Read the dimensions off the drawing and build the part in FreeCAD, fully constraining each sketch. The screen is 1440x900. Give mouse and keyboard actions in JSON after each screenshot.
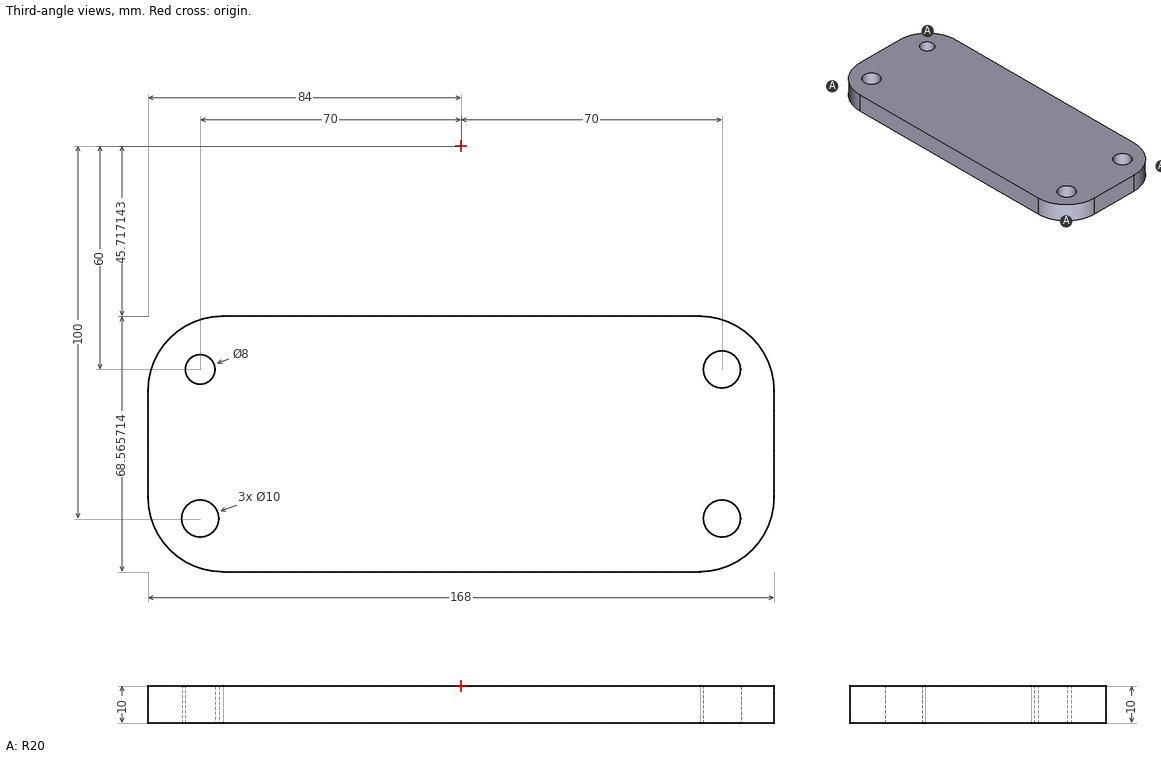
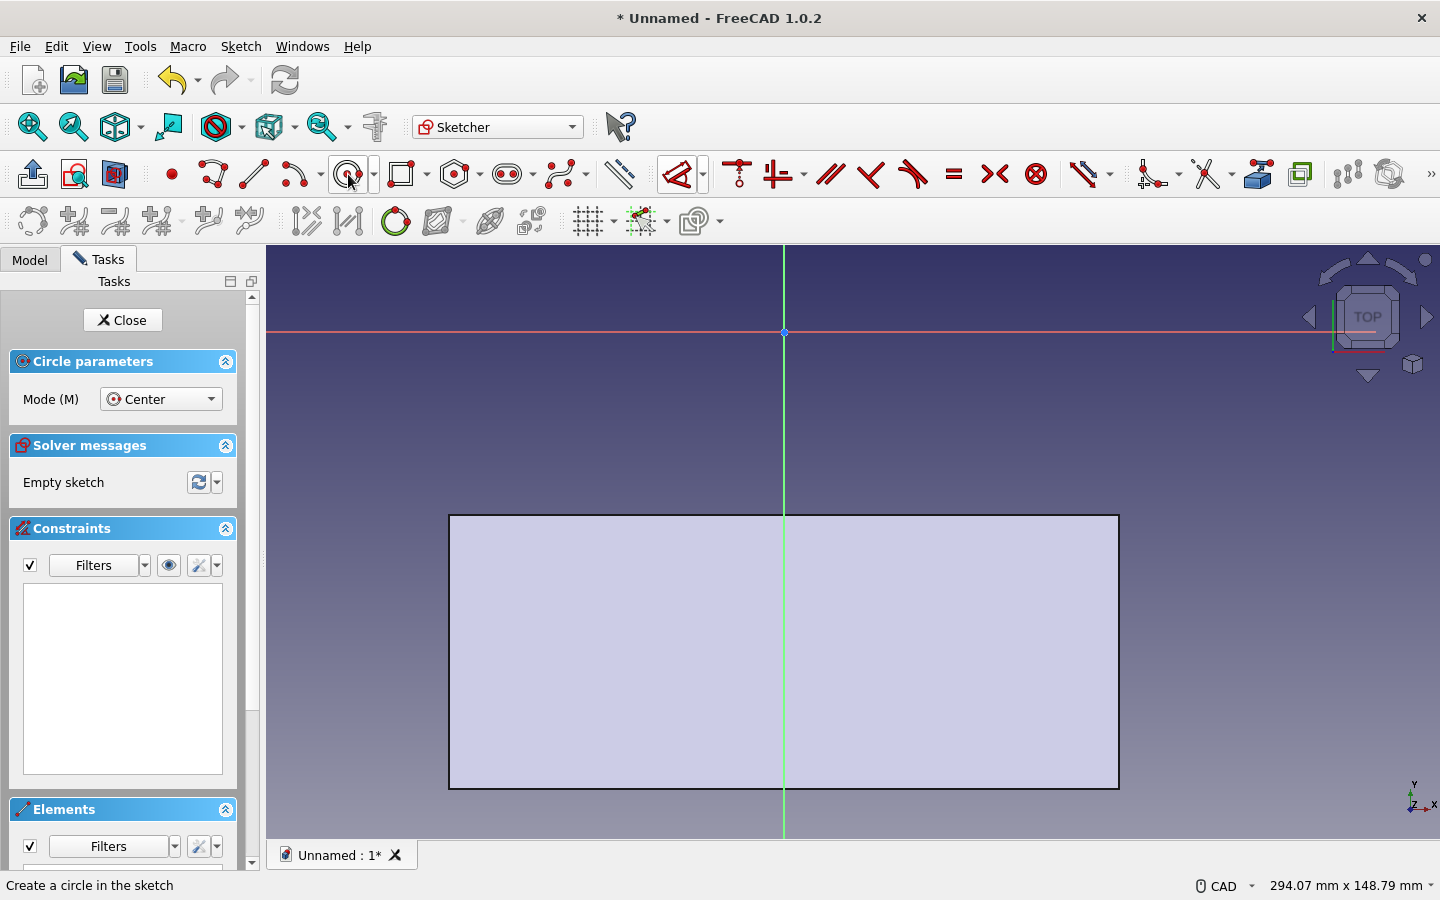
{"action": "scroll", "coordinate": [505, 572], "scroll_direction": "up", "scroll_amount": 2}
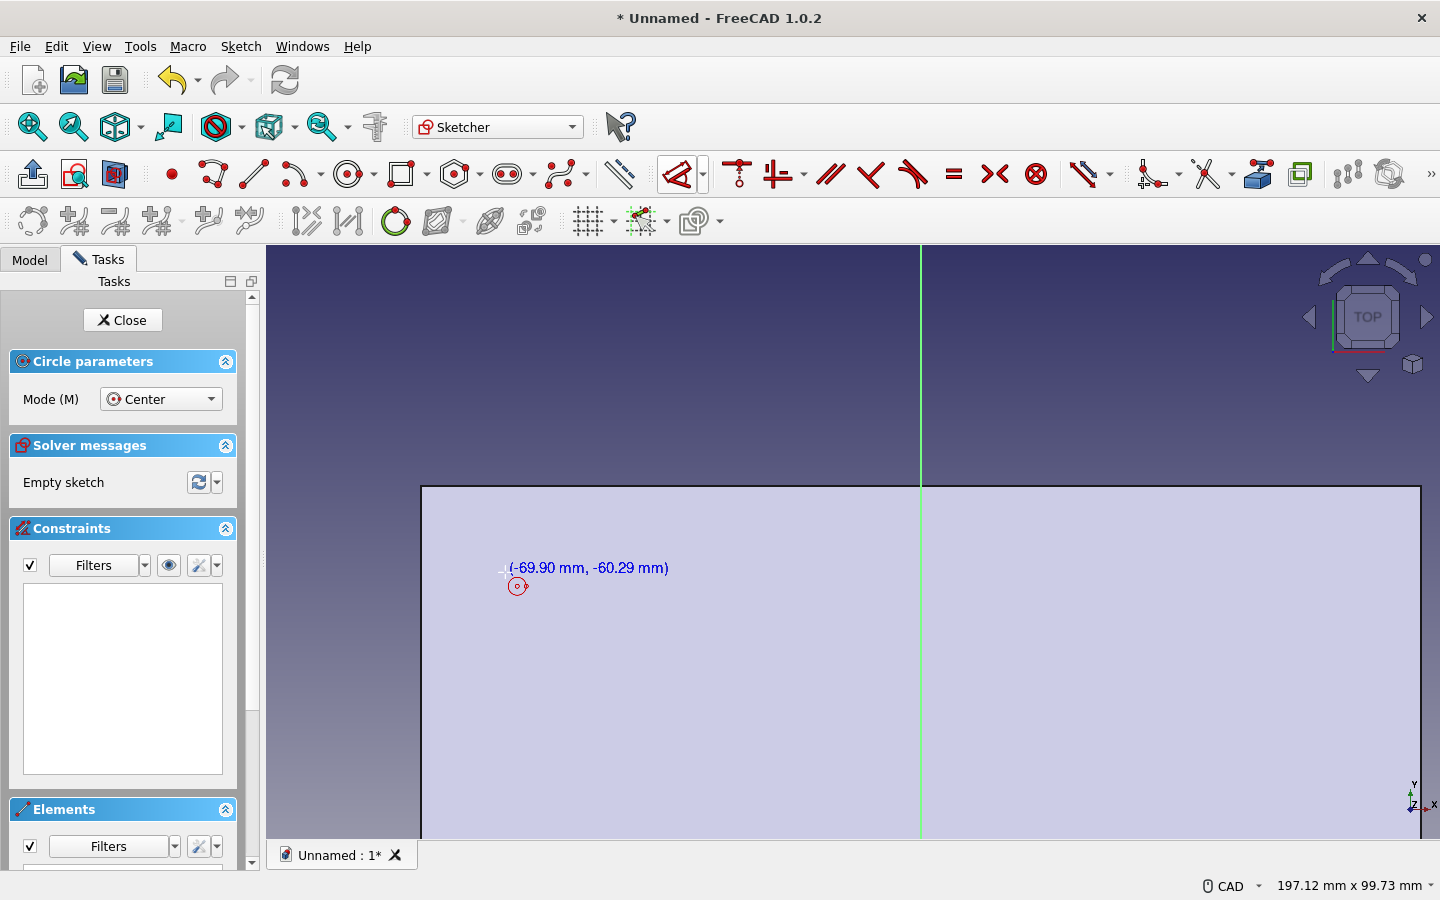
{"action": "left_click", "coordinate": [504, 572]}
{"action": "left_click", "coordinate": [521, 555]}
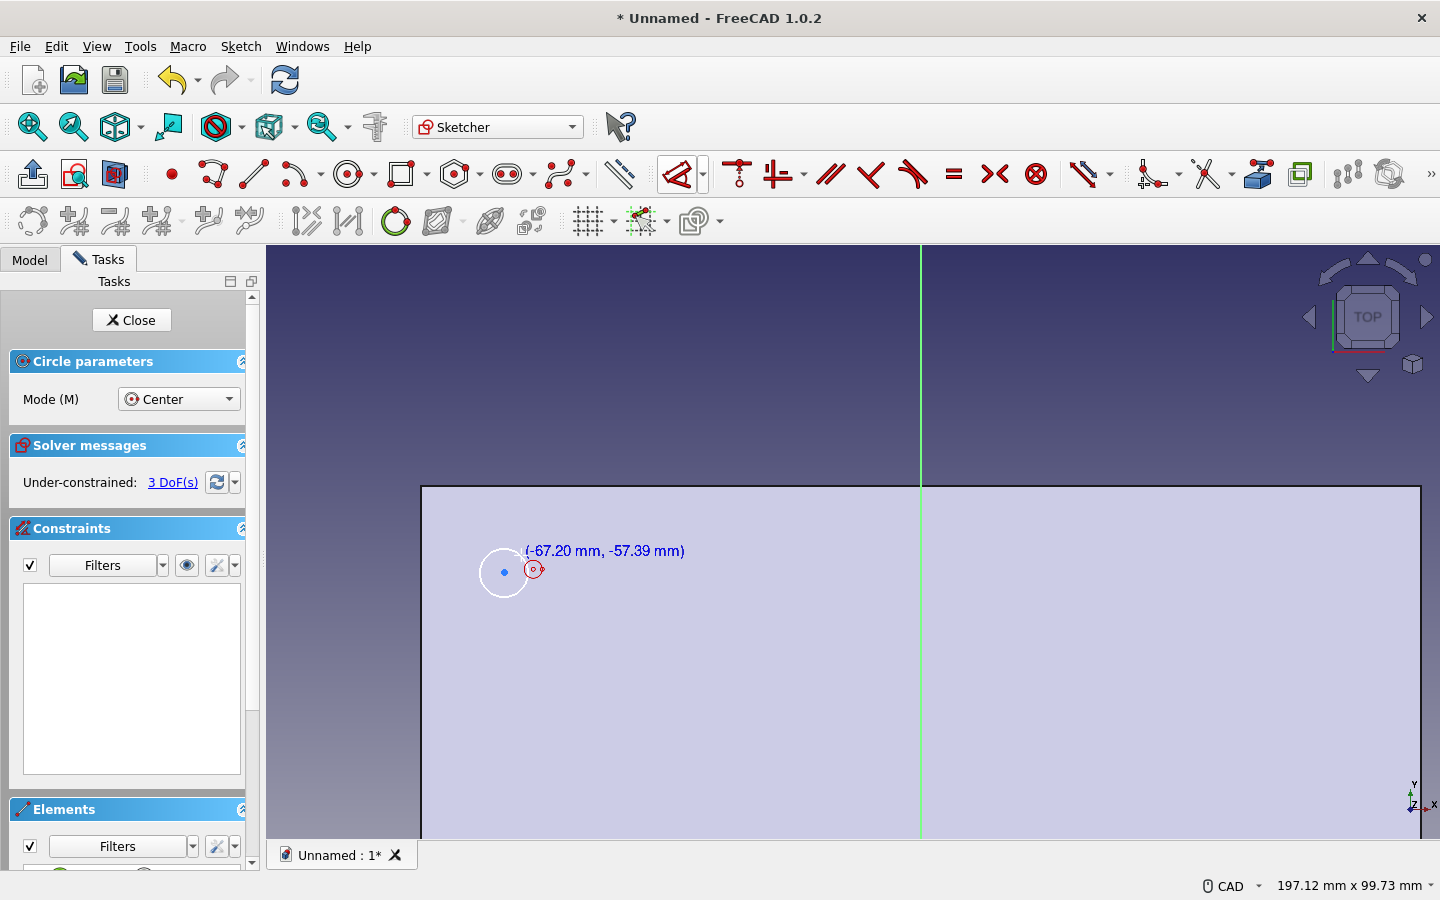
{"action": "left_click", "coordinate": [504, 810]}
{"action": "left_click", "coordinate": [525, 789]}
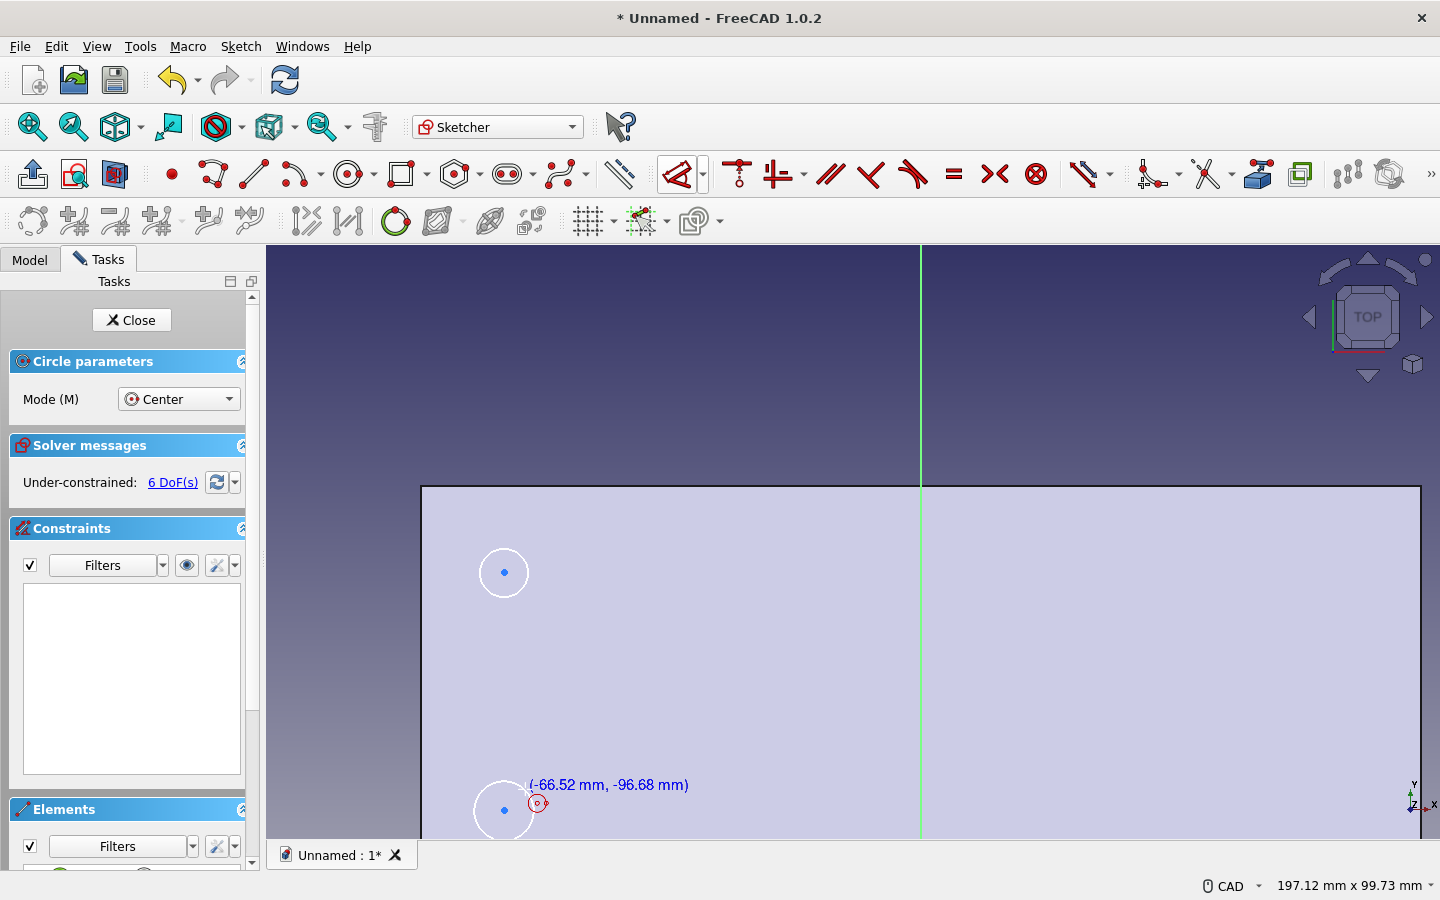
{"action": "scroll", "coordinate": [507, 573], "scroll_direction": "down", "scroll_amount": 2}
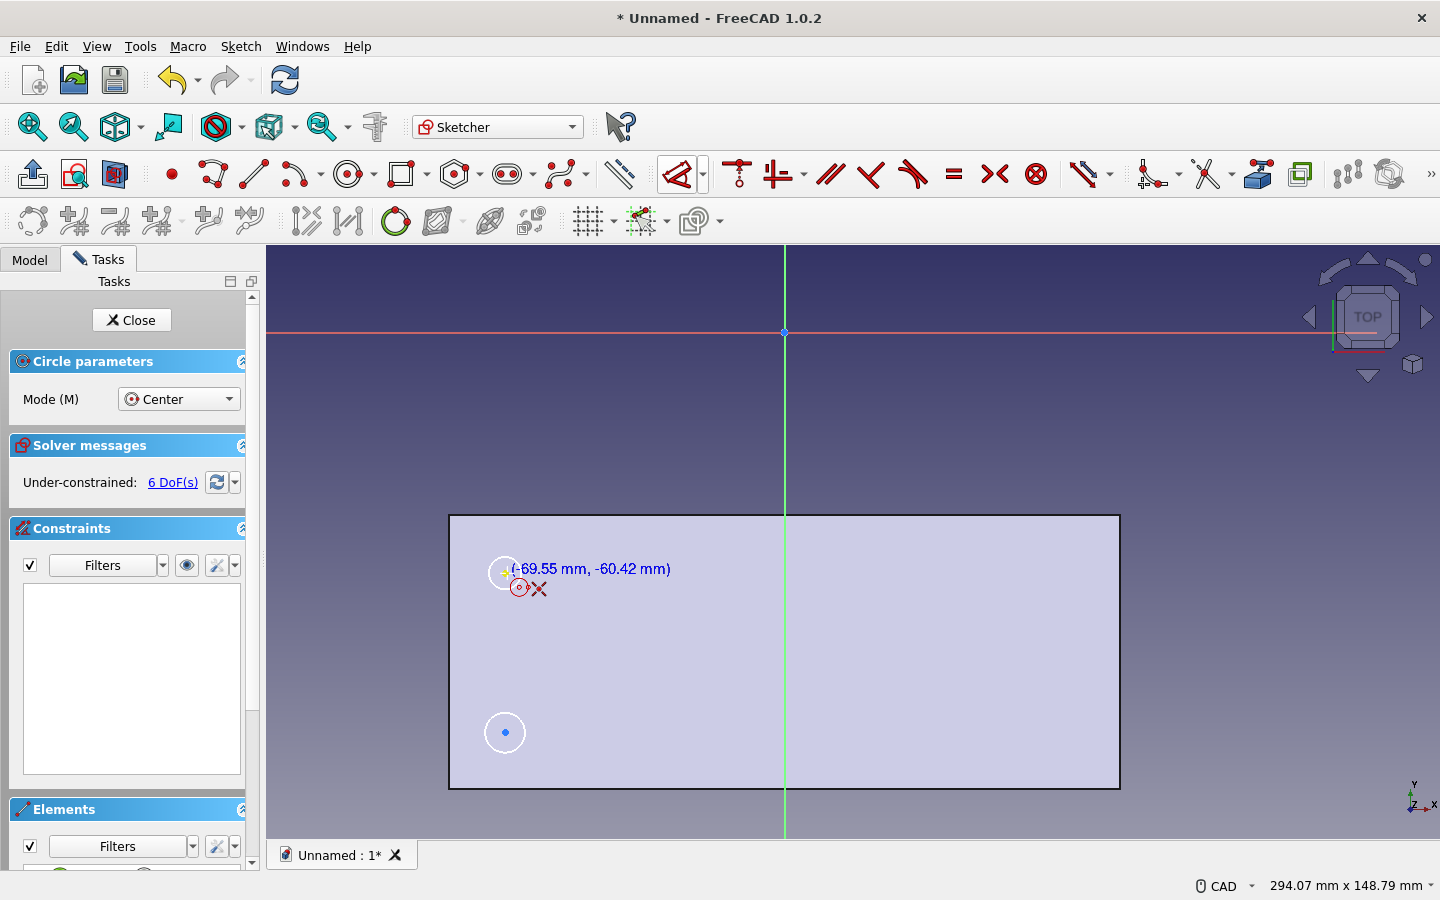
{"action": "left_click", "coordinate": [1064, 572]}
{"action": "left_click", "coordinate": [1078, 558]}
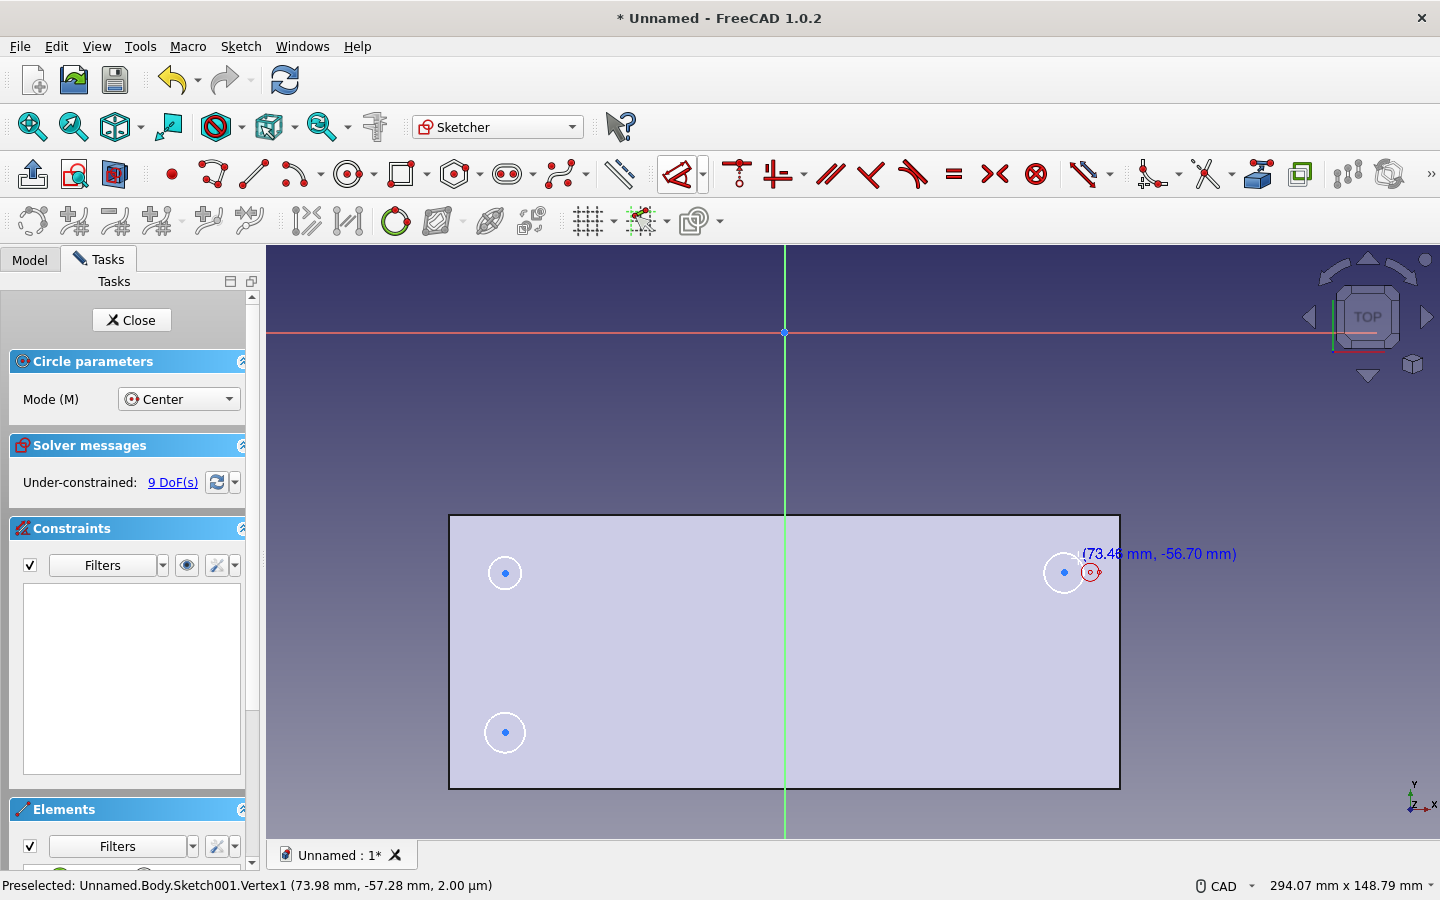
{"action": "left_click", "coordinate": [1064, 732]}
{"action": "left_click", "coordinate": [1078, 718]}
{"action": "key", "text": "Escape"}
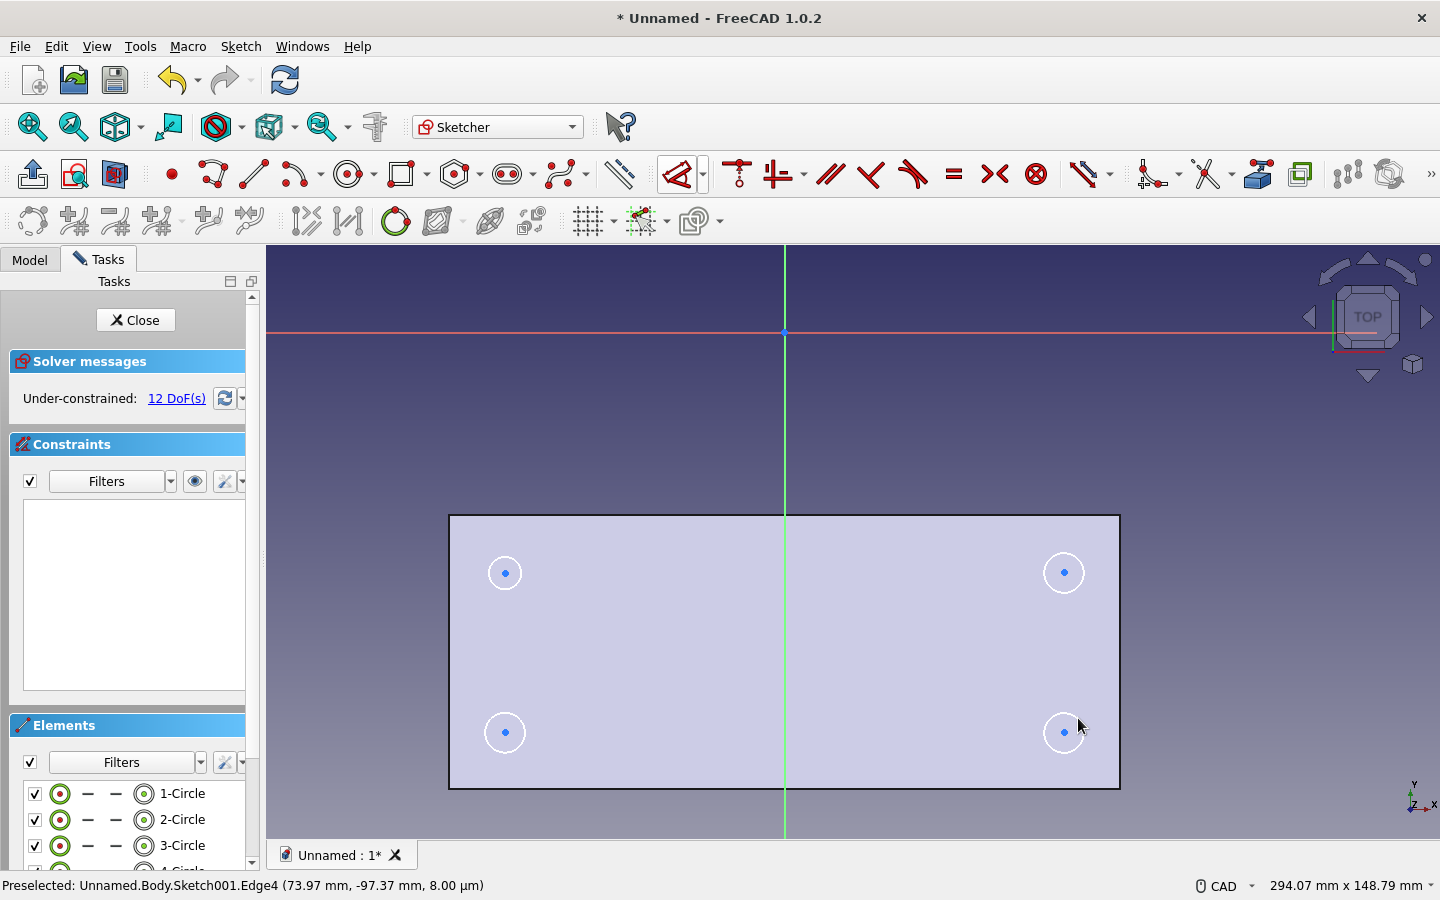
{"action": "left_click", "coordinate": [519, 719]}